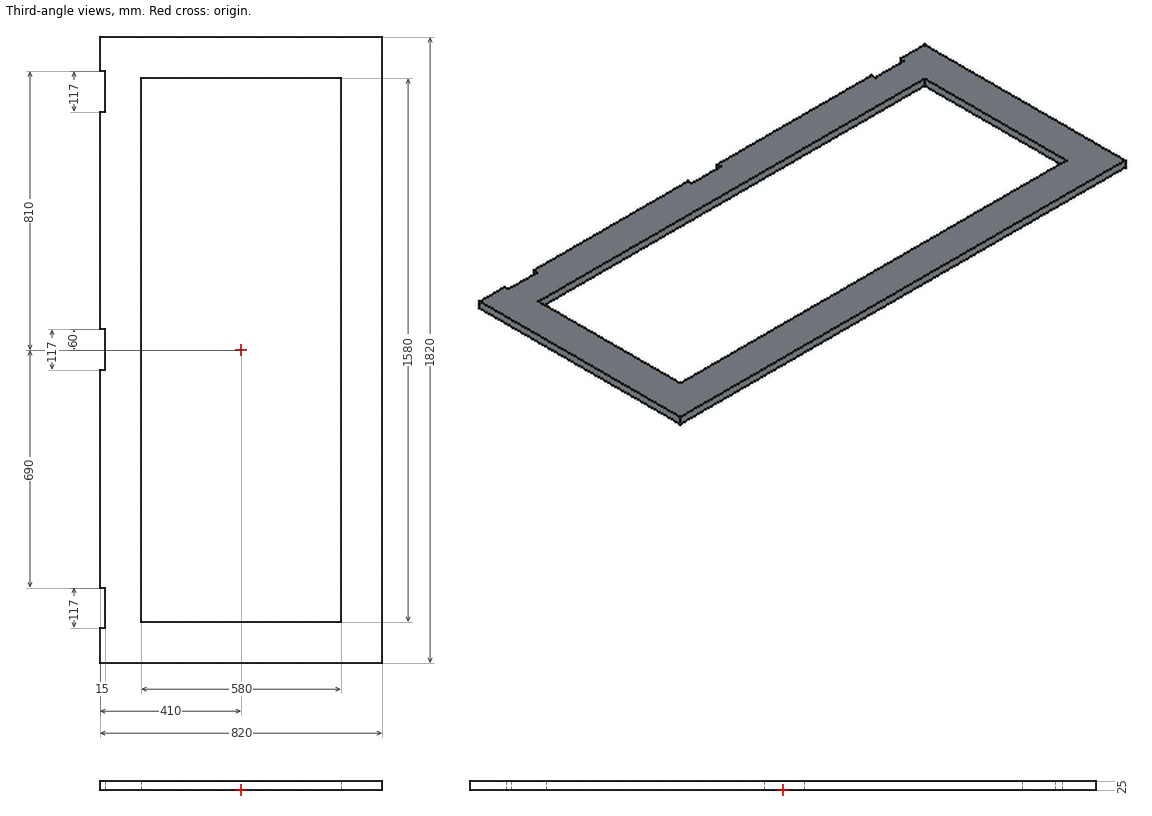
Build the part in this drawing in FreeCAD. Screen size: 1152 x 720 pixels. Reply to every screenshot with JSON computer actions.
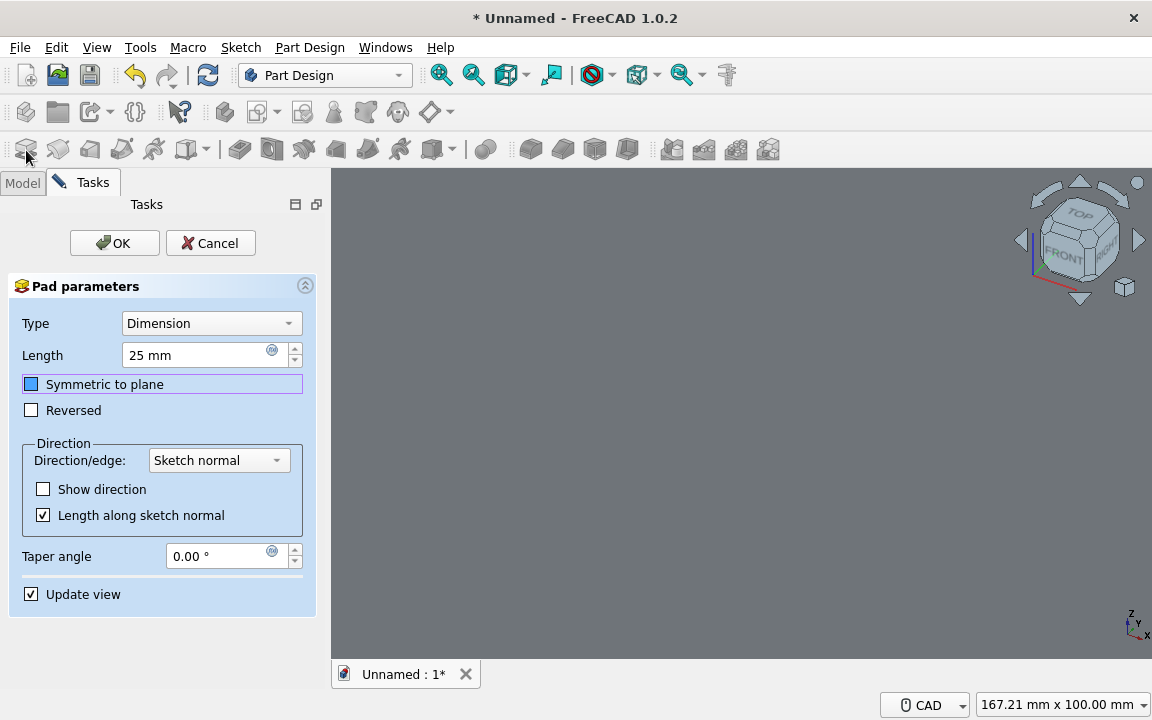
{"action": "left_click", "coordinate": [115, 243]}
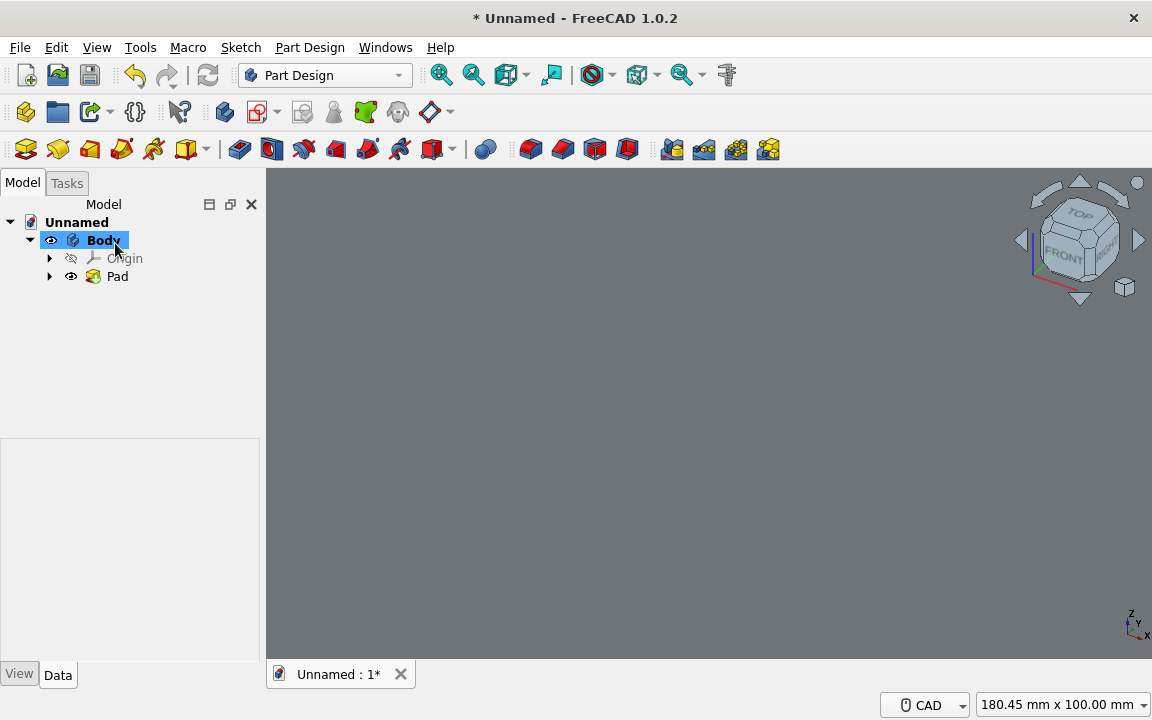
{"action": "left_click", "coordinate": [442, 76]}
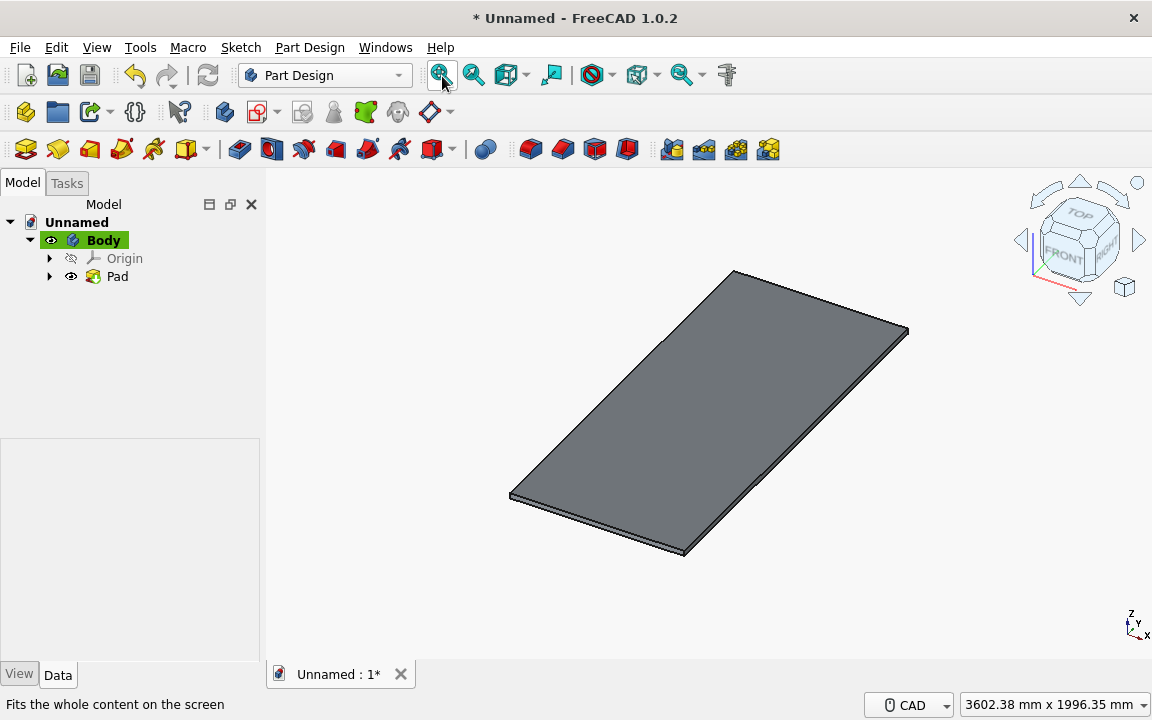
{"action": "left_click", "coordinate": [741, 378]}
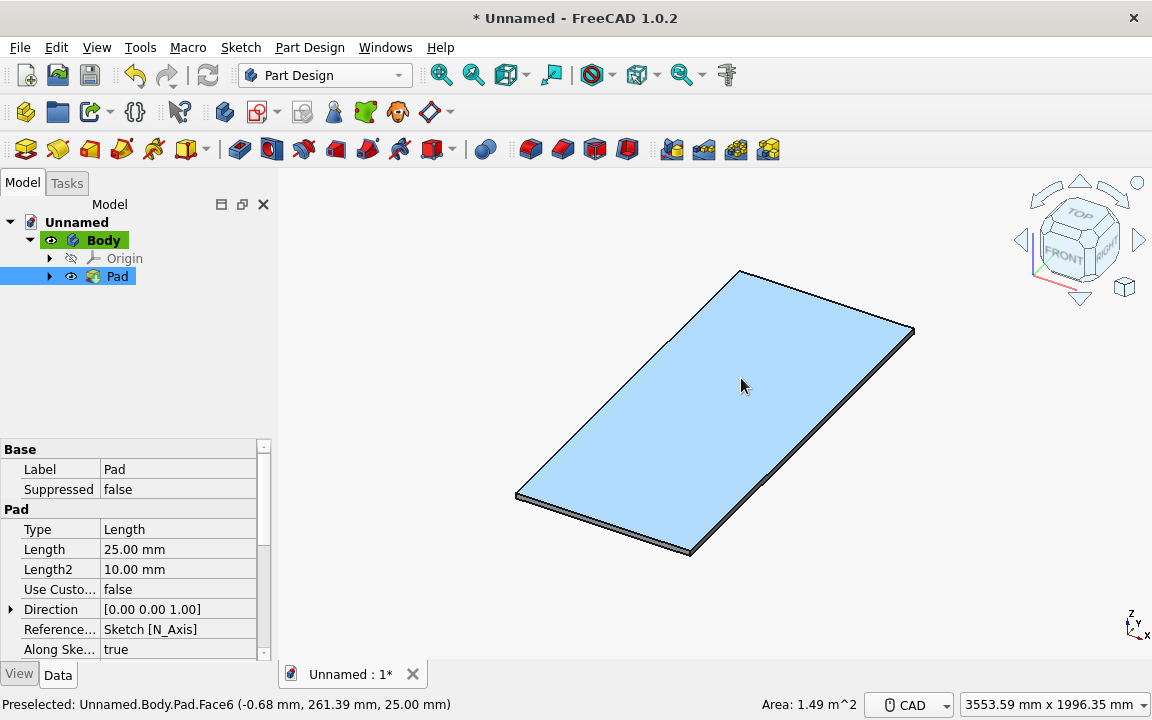
{"action": "left_click", "coordinate": [258, 112]}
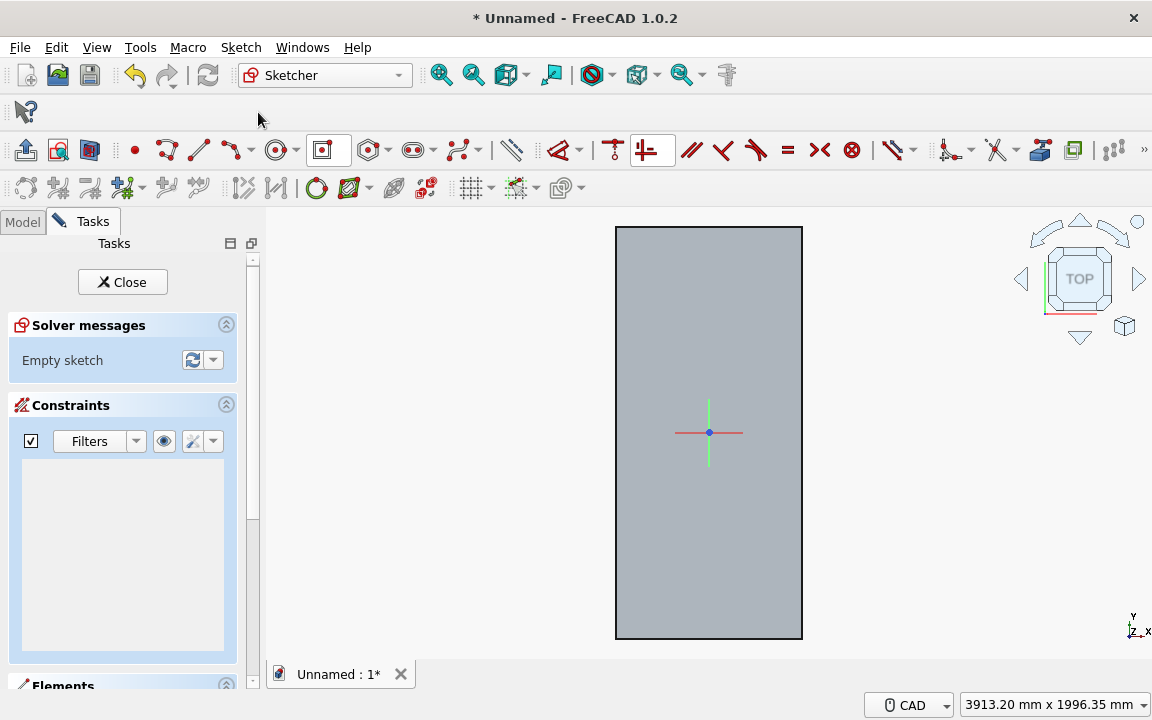
{"action": "scroll", "coordinate": [331, 433], "scroll_direction": "down", "scroll_amount": 1}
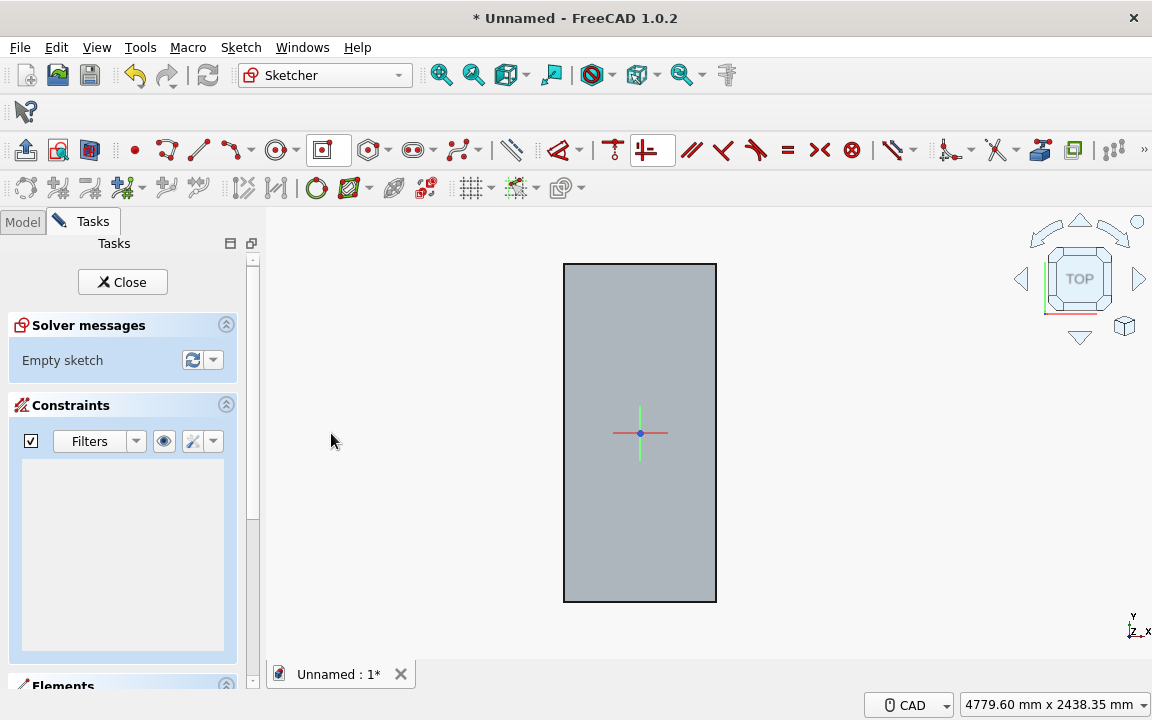
{"action": "left_click", "coordinate": [322, 150]}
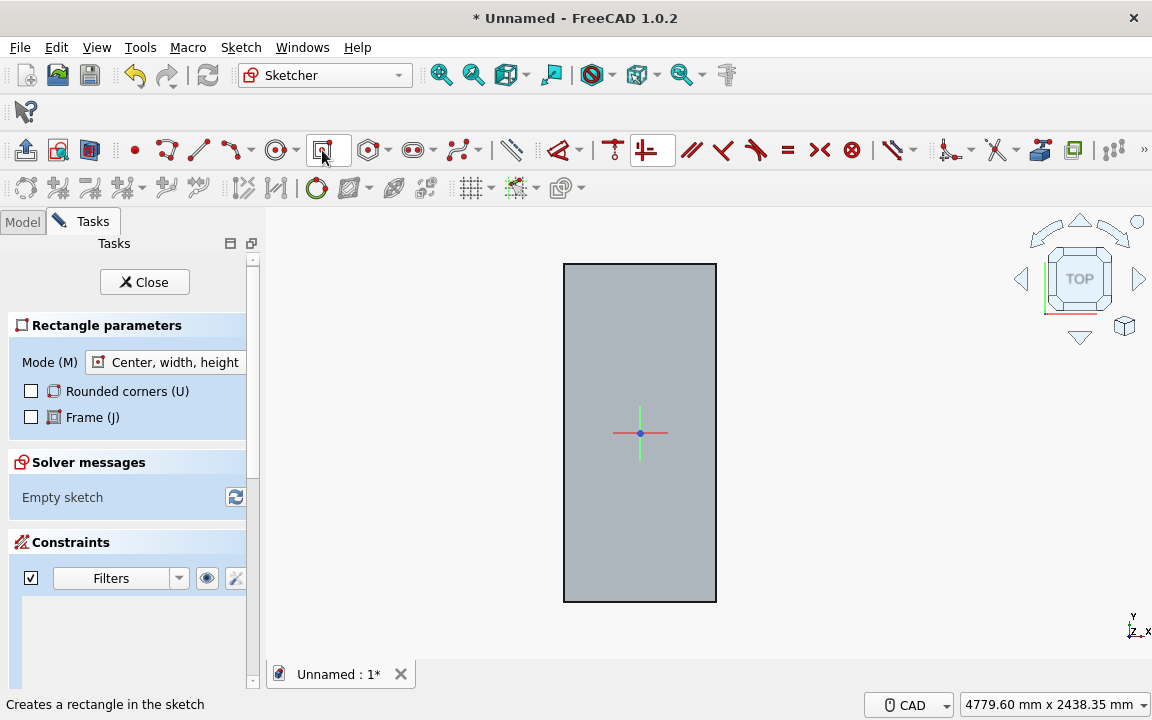
{"action": "left_click", "coordinate": [640, 433]}
{"action": "mouse_move", "coordinate": [694, 287]}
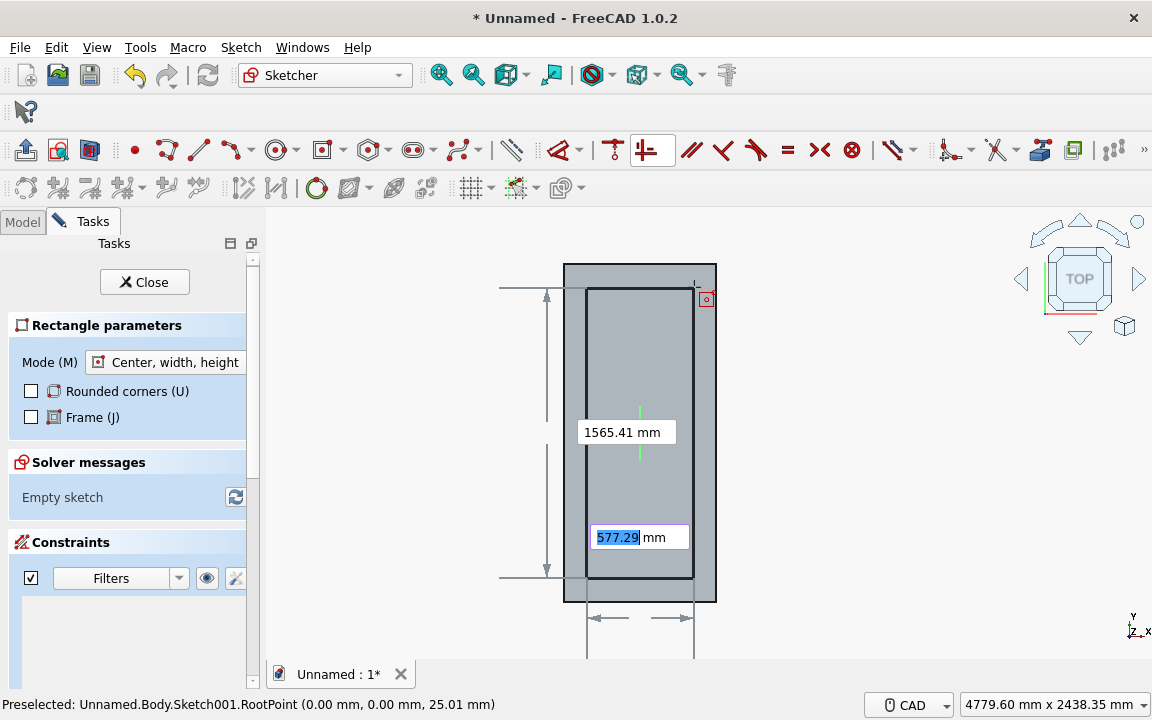
{"action": "type", "text": "580"}
{"action": "key", "text": "Tab"}
{"action": "type", "text": "1580"}
{"action": "key", "text": "Return"}
{"action": "key", "text": "Escape"}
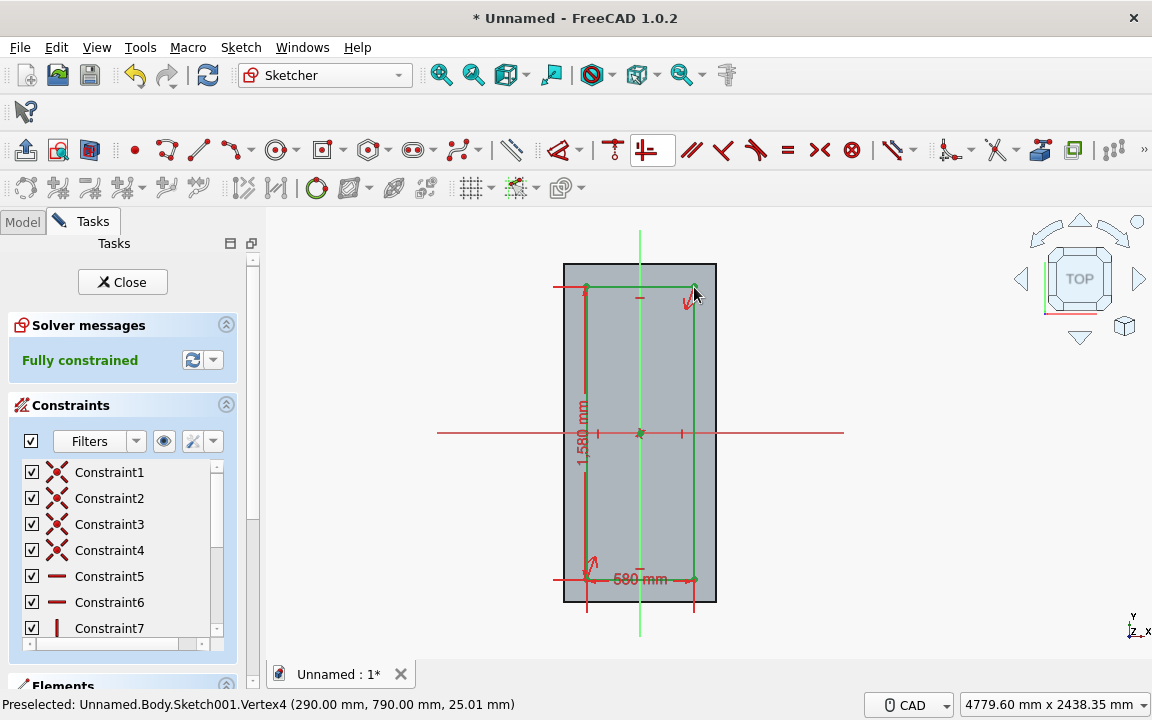
{"action": "left_click", "coordinate": [123, 282]}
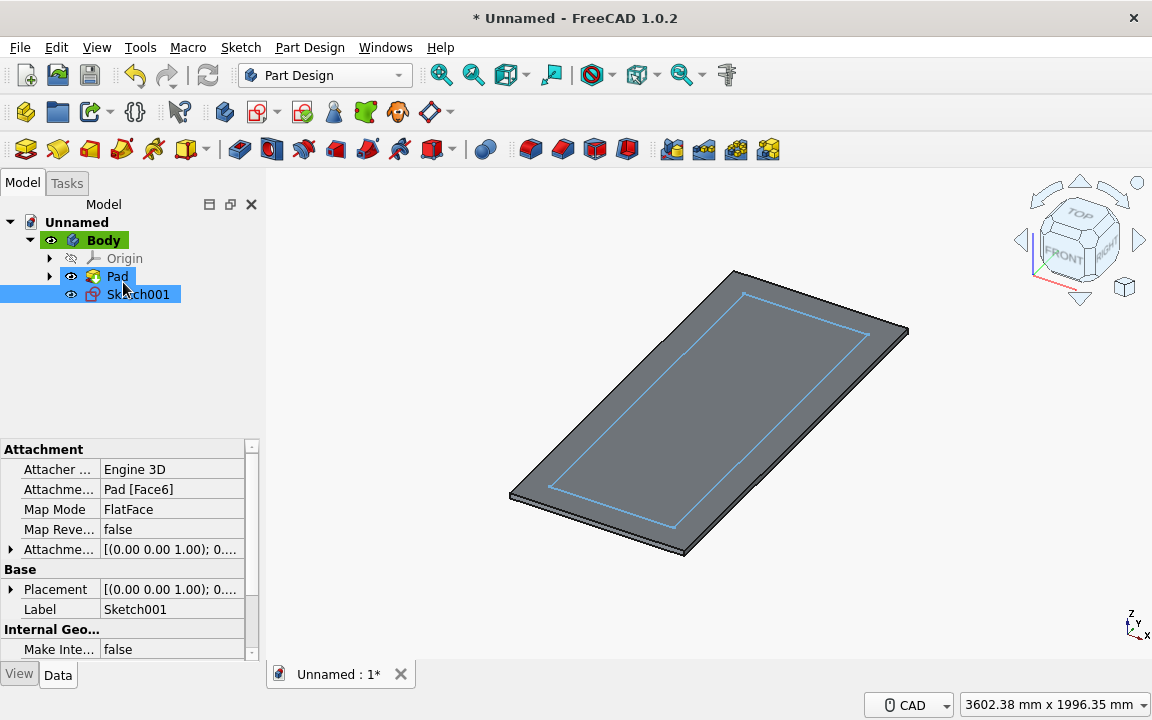
{"action": "left_click", "coordinate": [240, 150]}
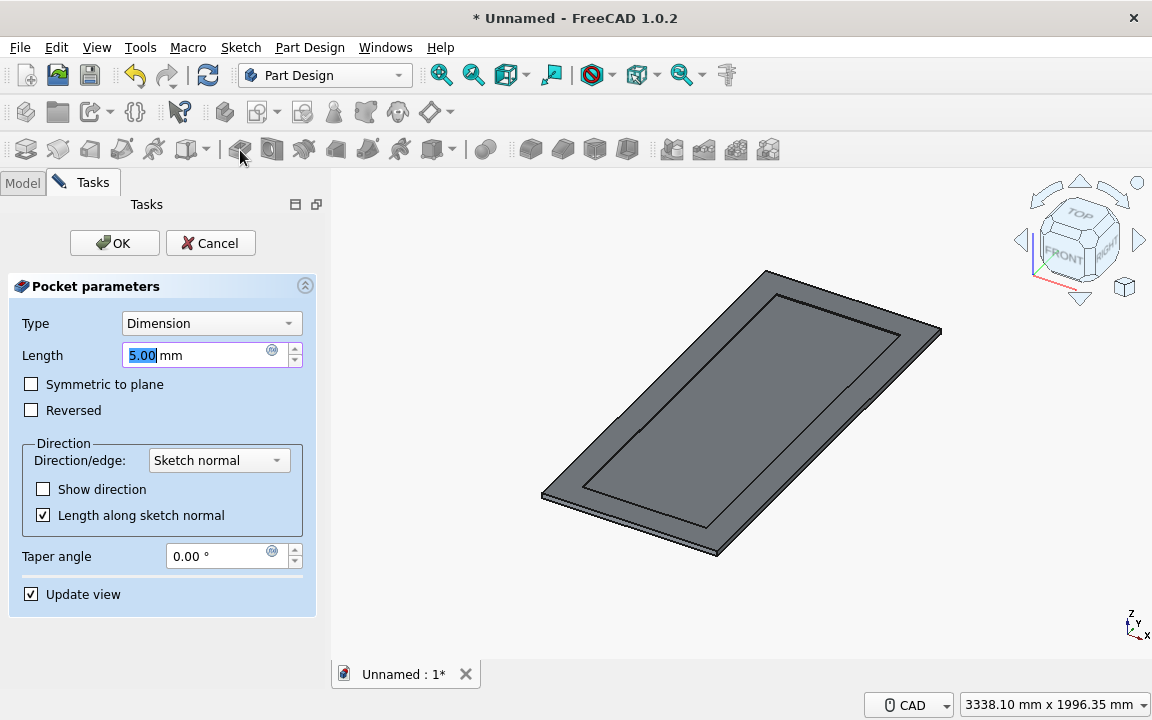
{"action": "left_click", "coordinate": [212, 324]}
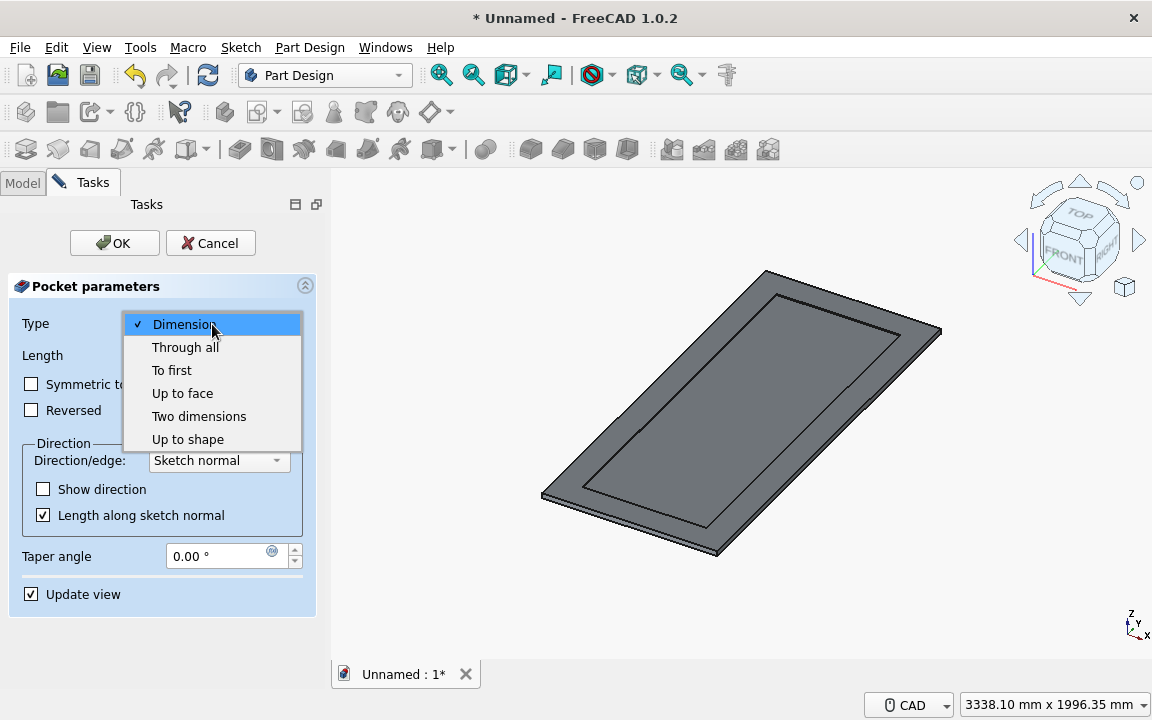
{"action": "left_click", "coordinate": [212, 348]}